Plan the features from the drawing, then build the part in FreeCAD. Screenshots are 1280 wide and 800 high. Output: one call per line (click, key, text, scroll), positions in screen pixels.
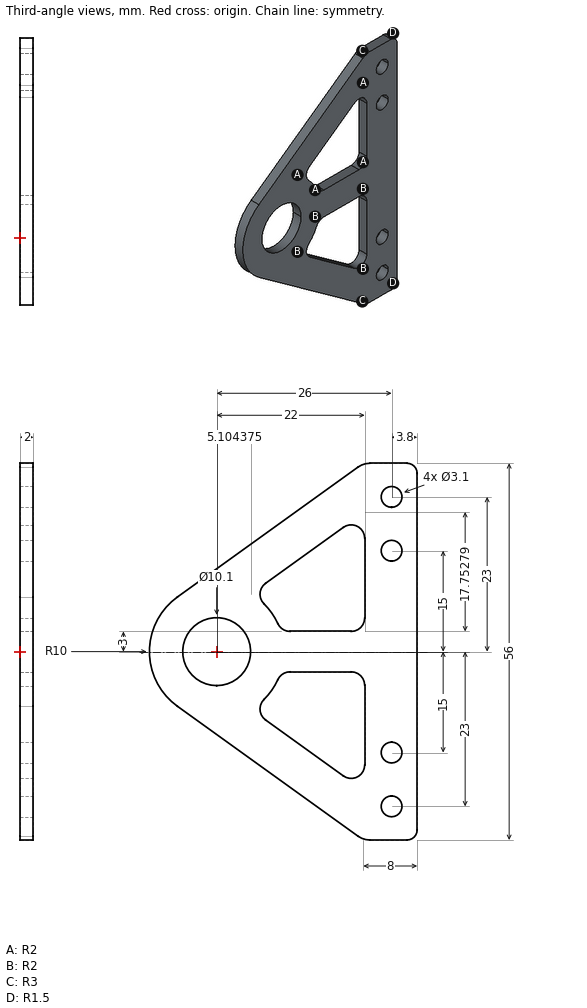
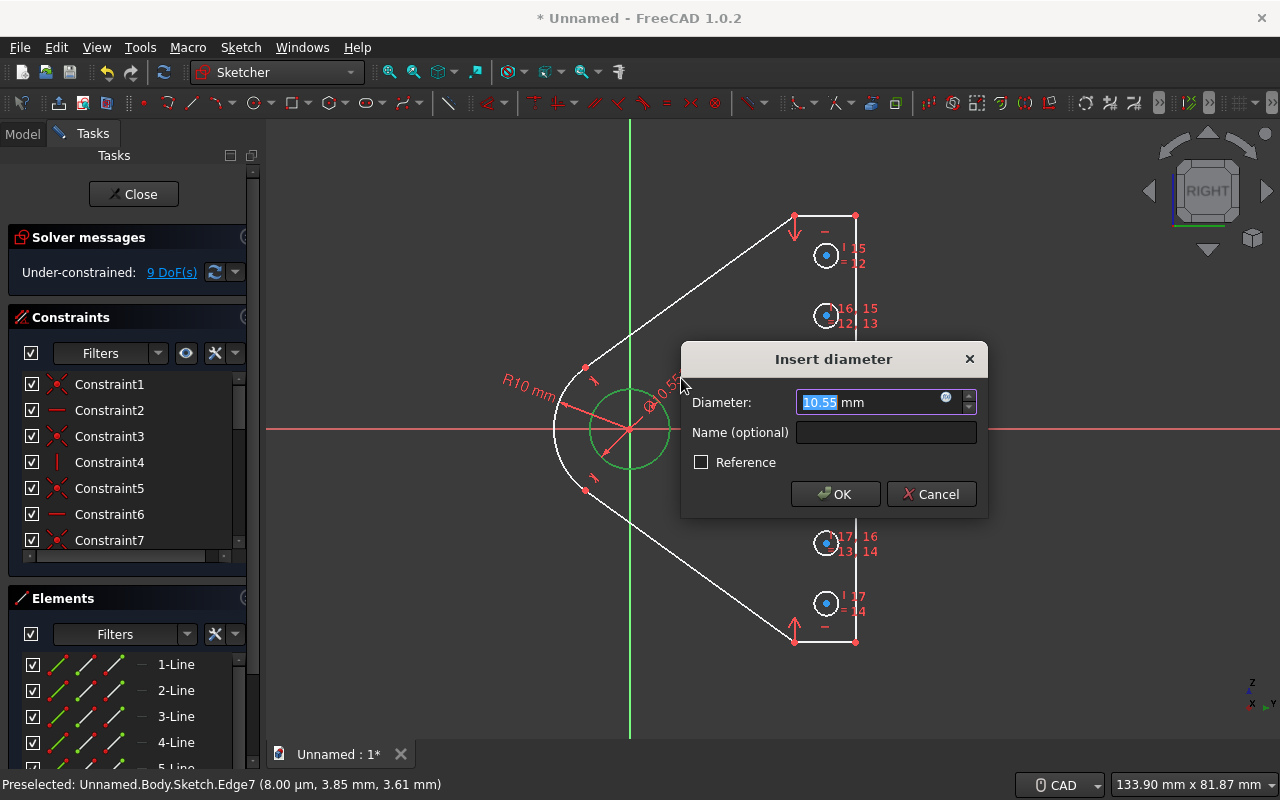
text(10.1)
key(Return)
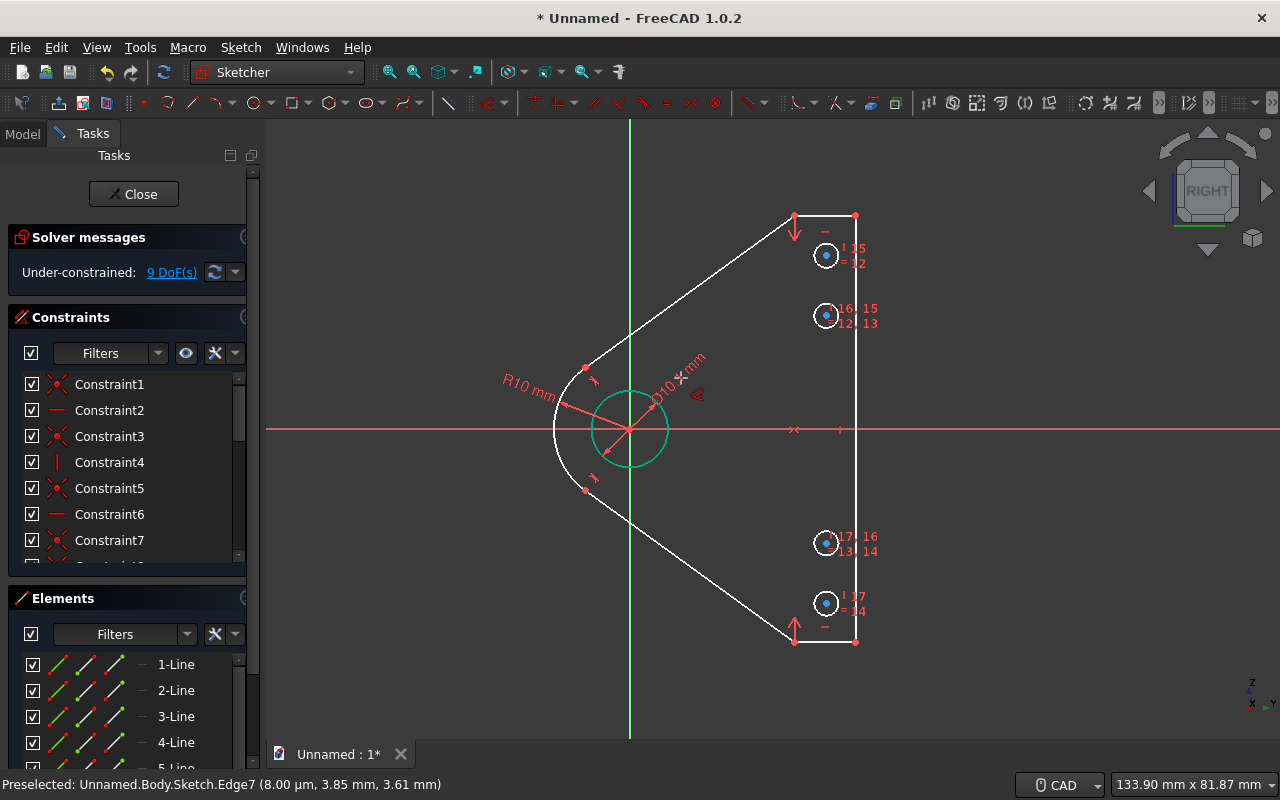
scroll(835, 247, up, 3)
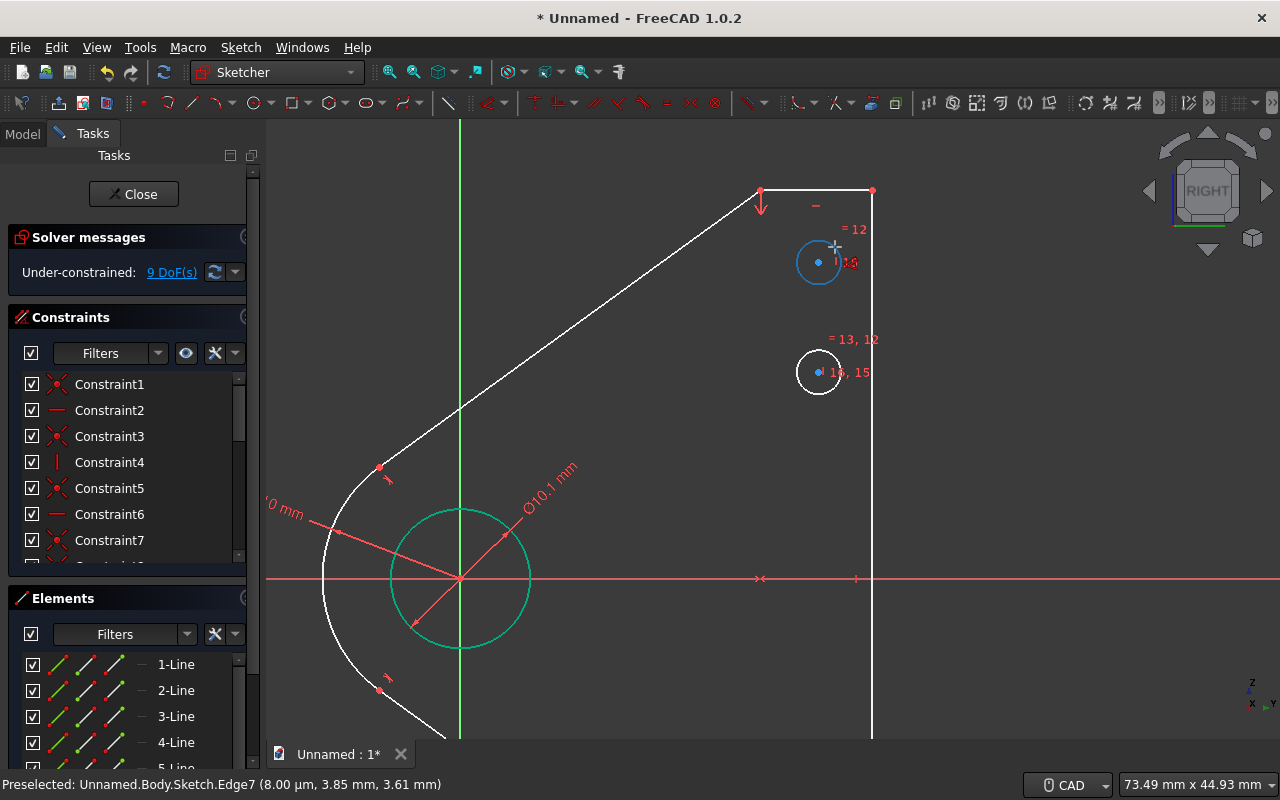
click(834, 247)
click(856, 224)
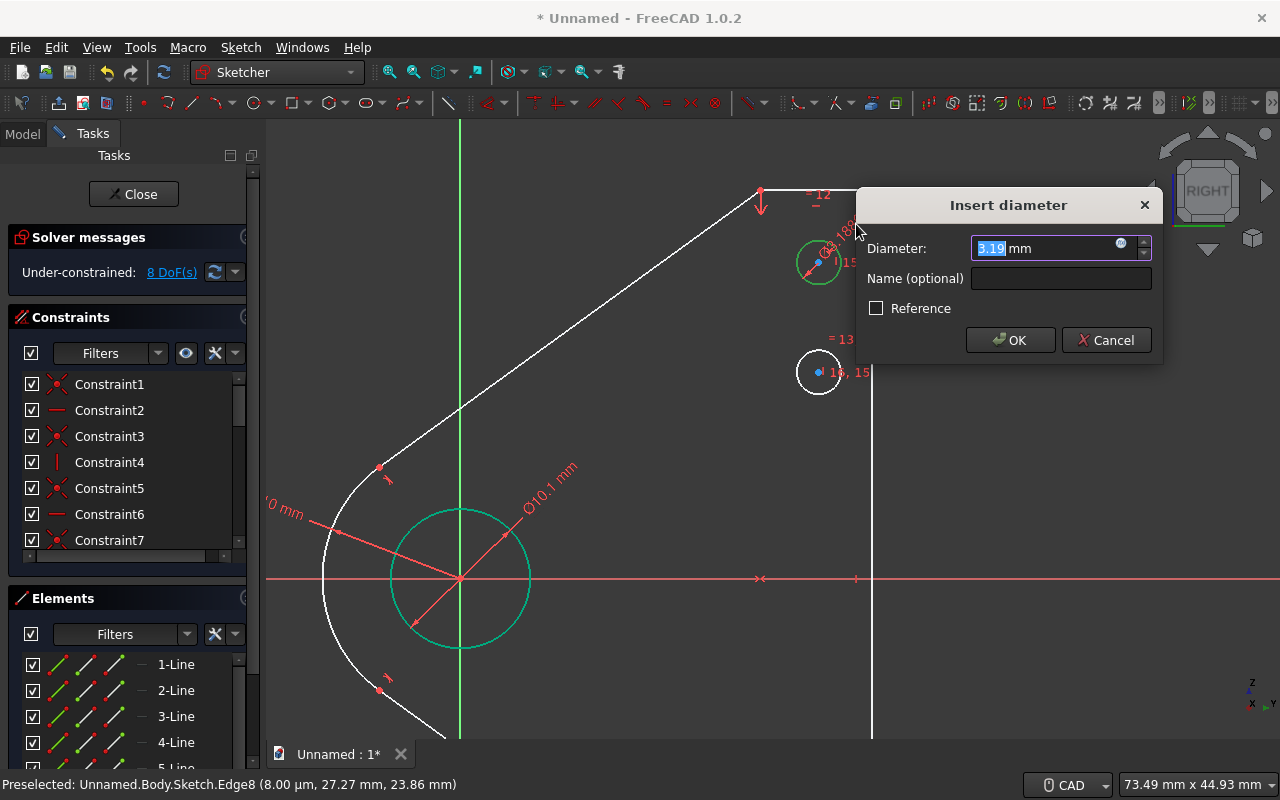
text(3.1)
key(Return)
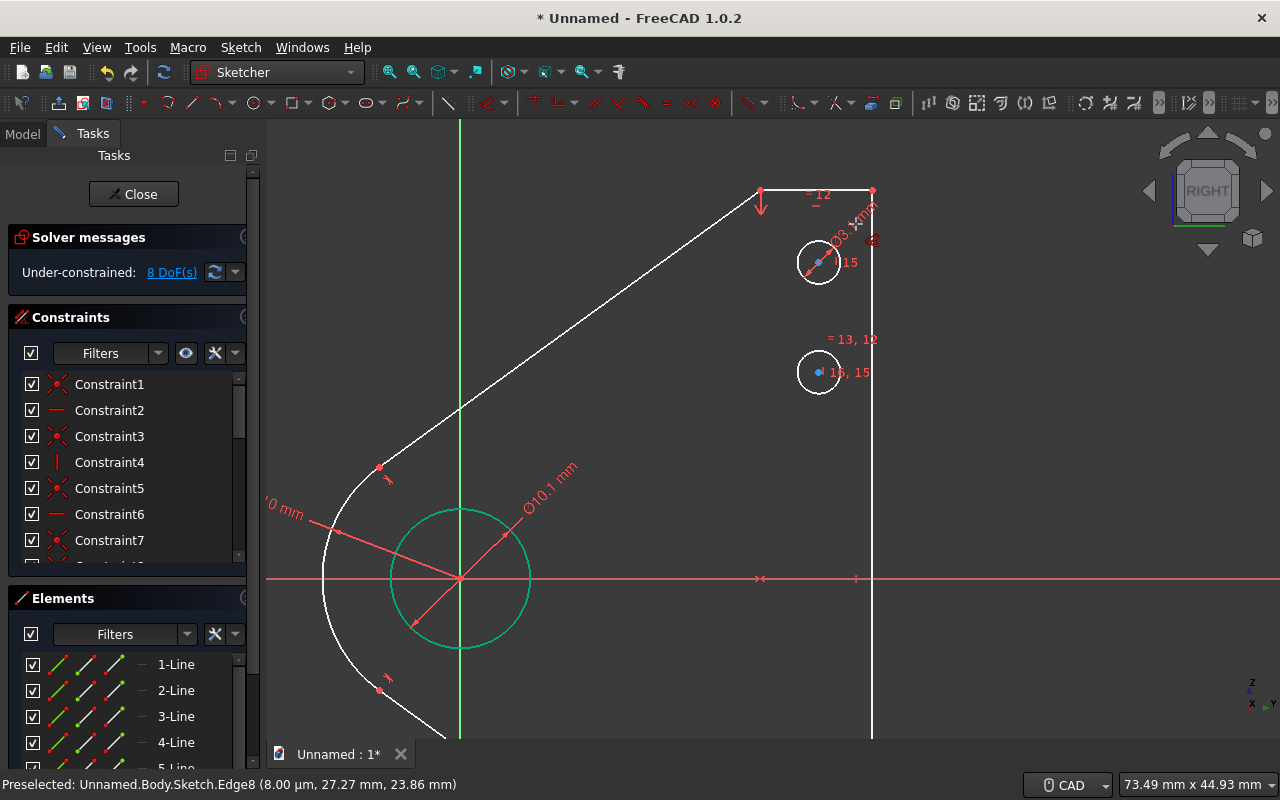
scroll(835, 247, down, 3)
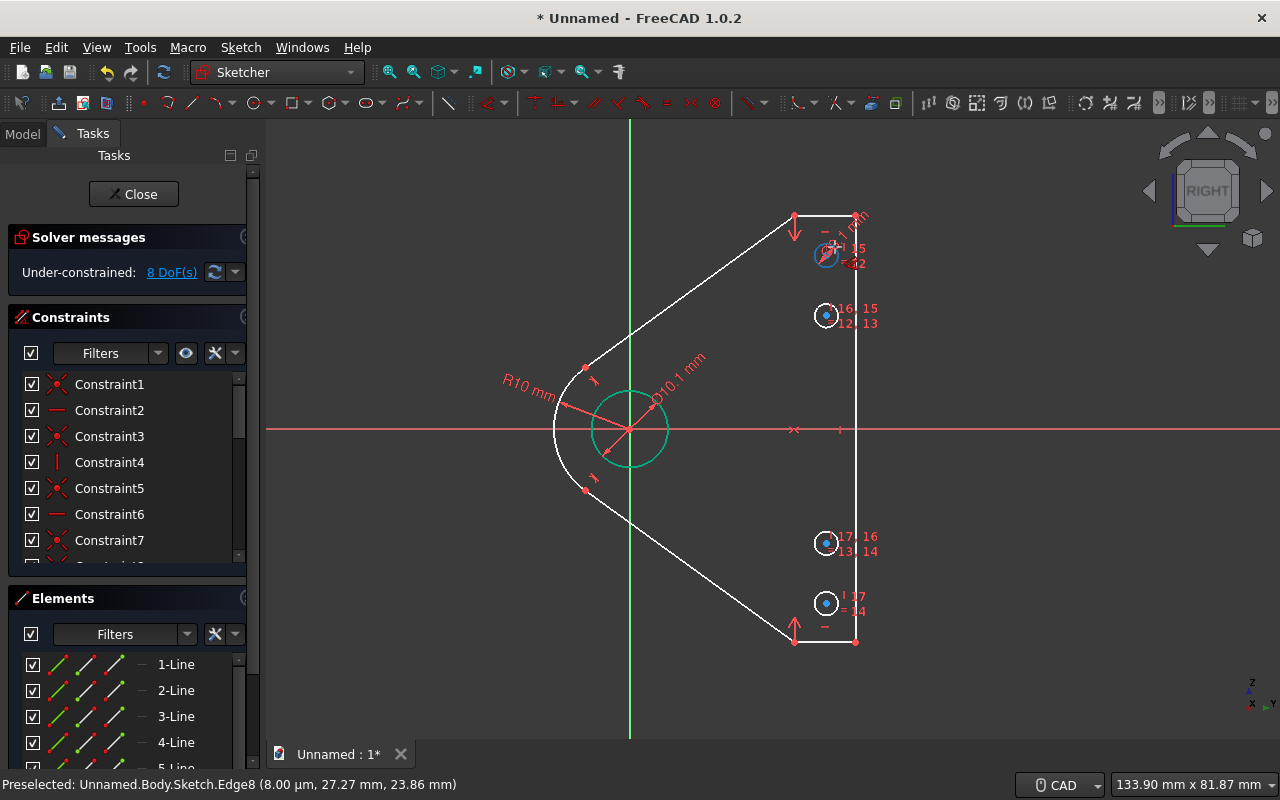
click(813, 642)
click(825, 676)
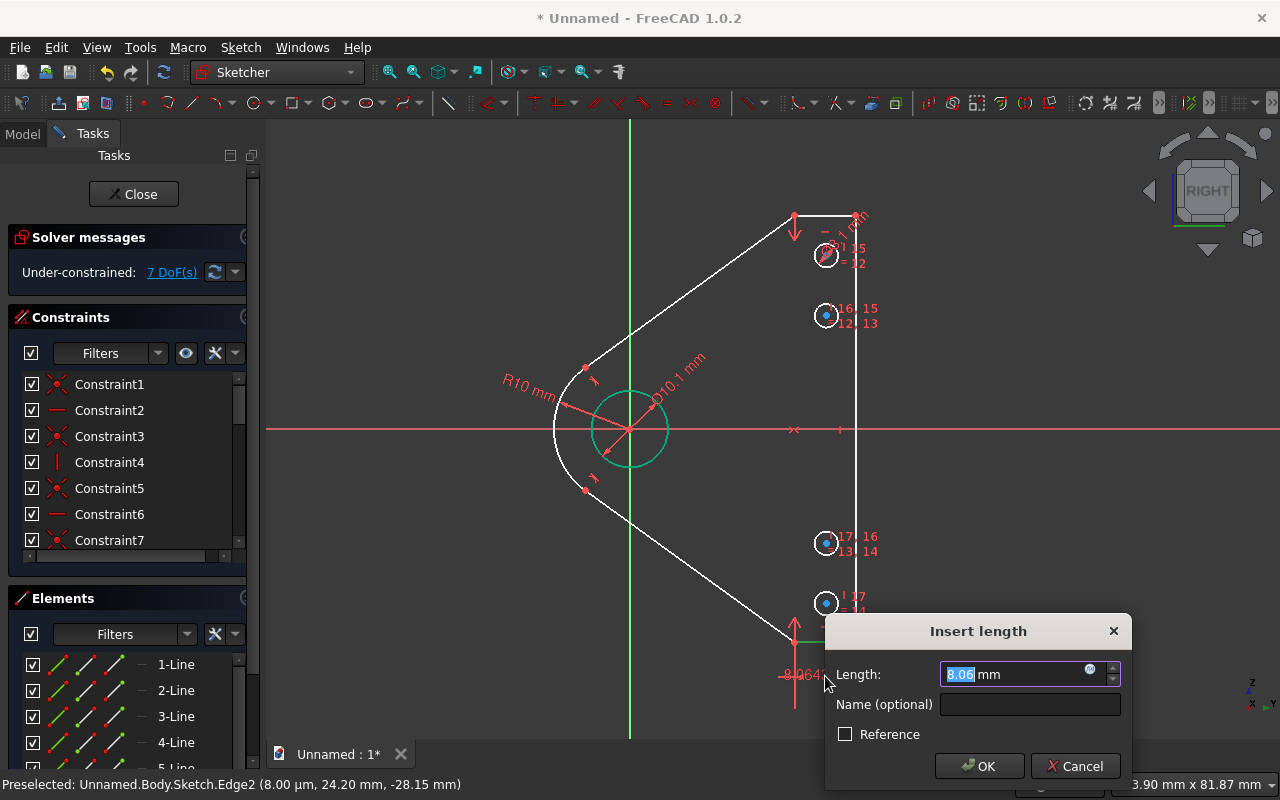
text(8)
key(Return)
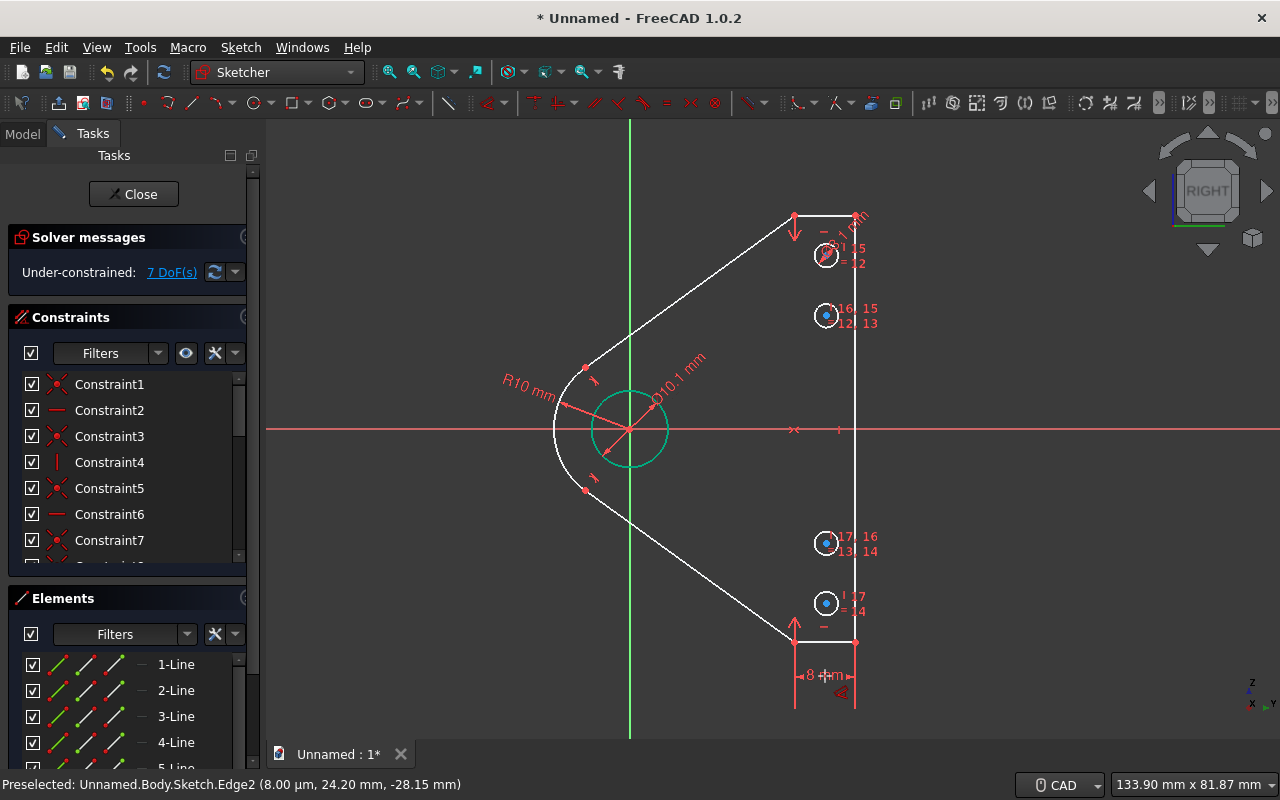
click(855, 514)
click(889, 331)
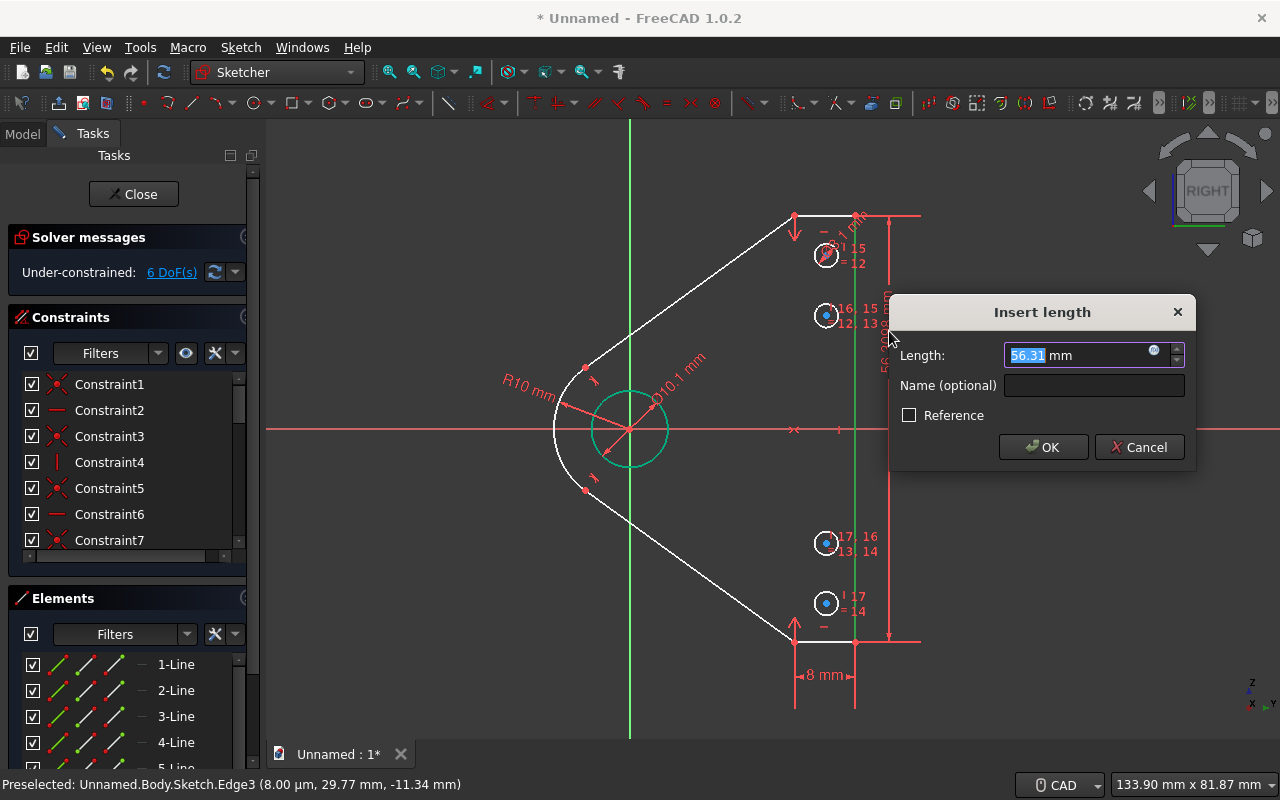
text(56)
key(Return)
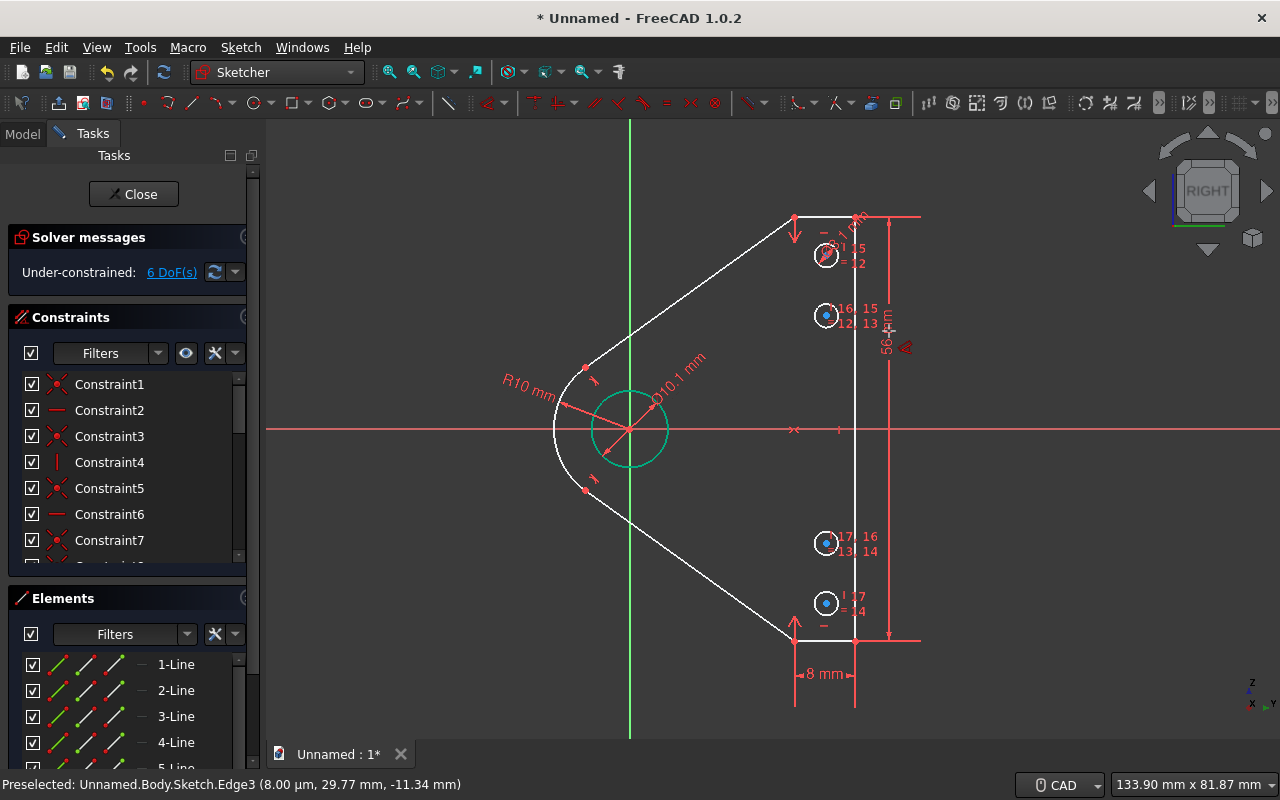
click(826, 256)
click(728, 222)